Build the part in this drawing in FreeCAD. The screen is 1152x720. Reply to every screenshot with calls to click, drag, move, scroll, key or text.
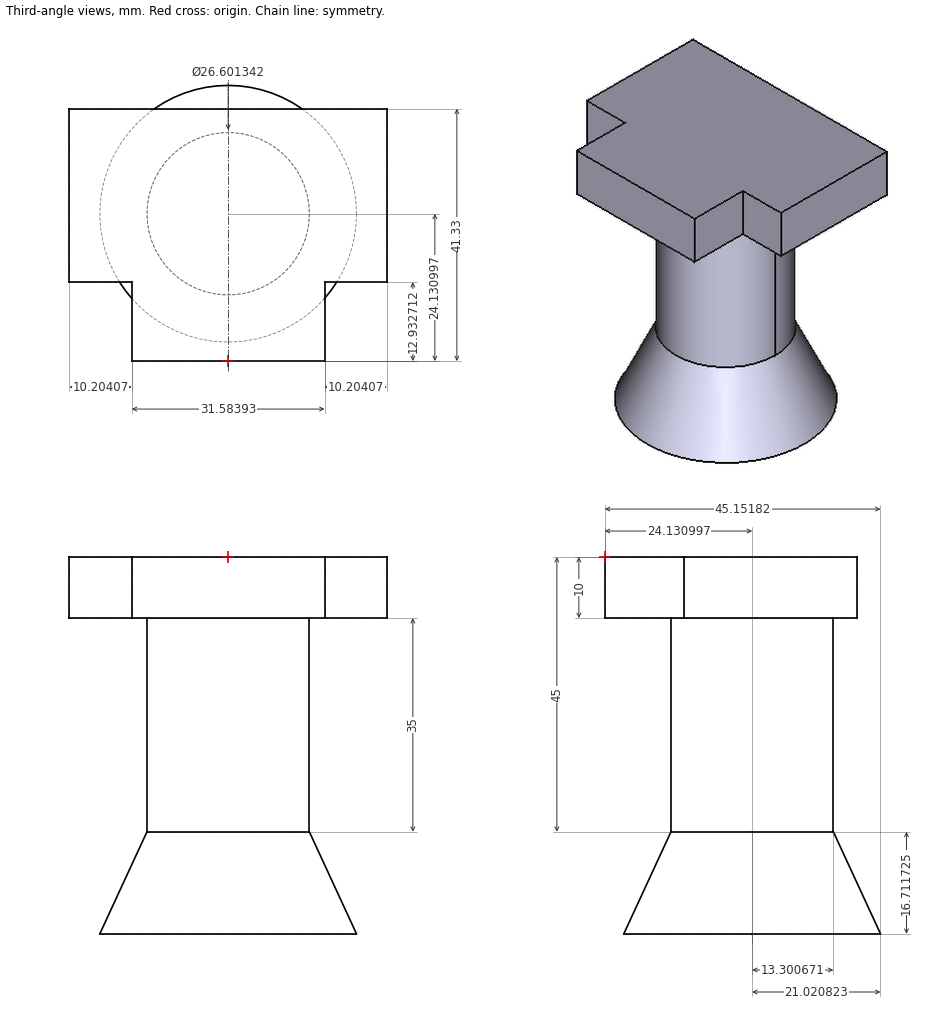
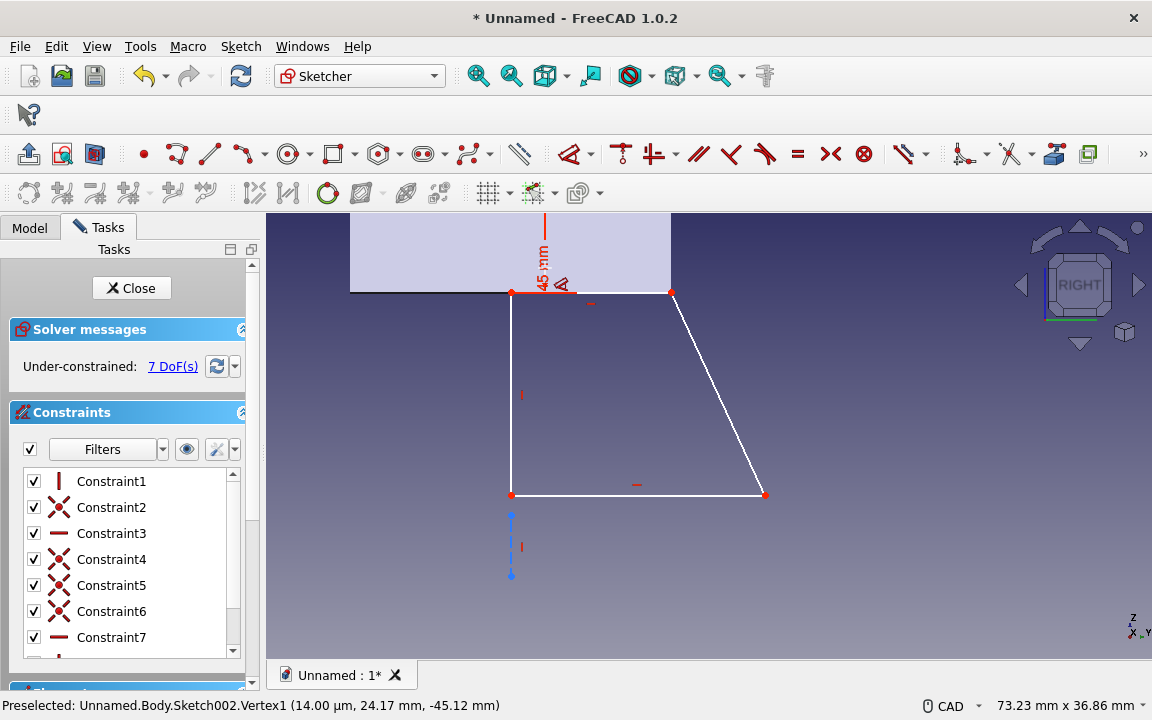
click(511, 354)
click(477, 394)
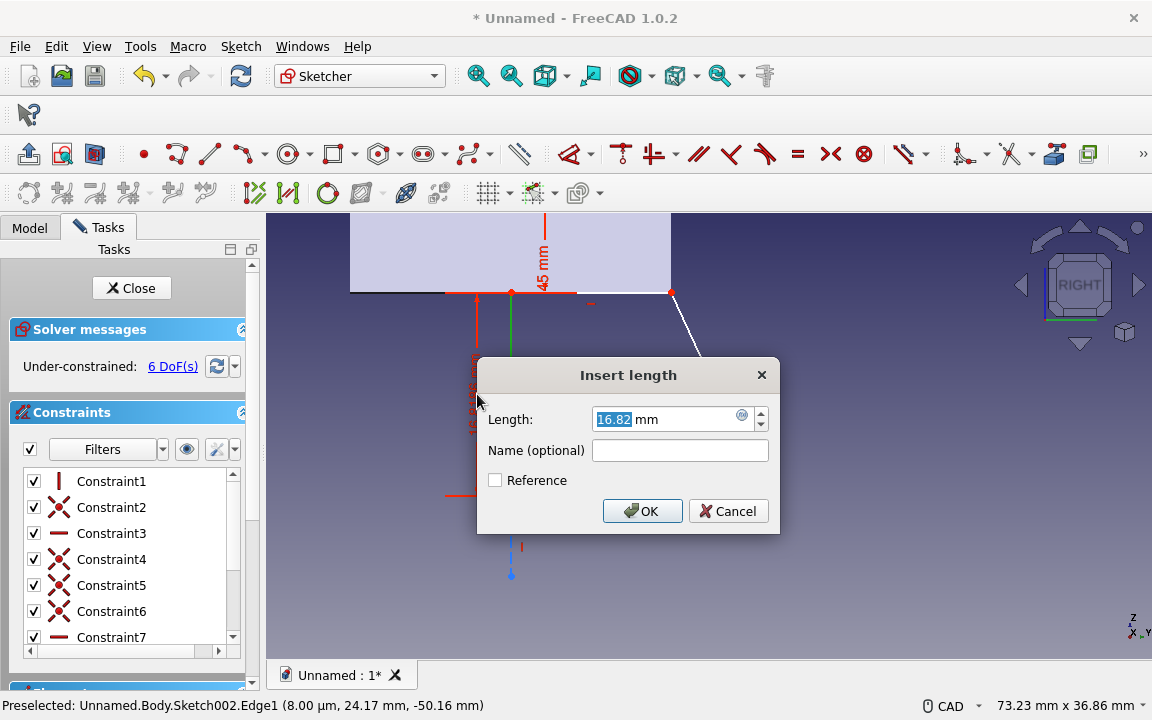
text(16.711725)
key(Return)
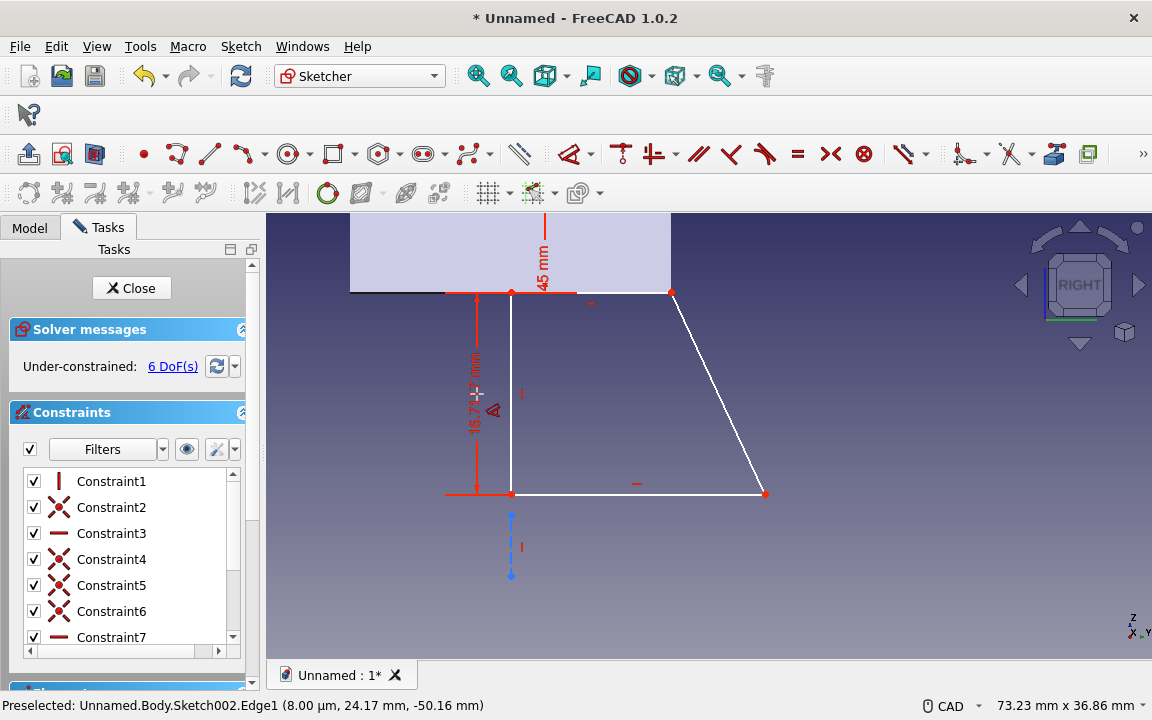
click(587, 495)
click(638, 529)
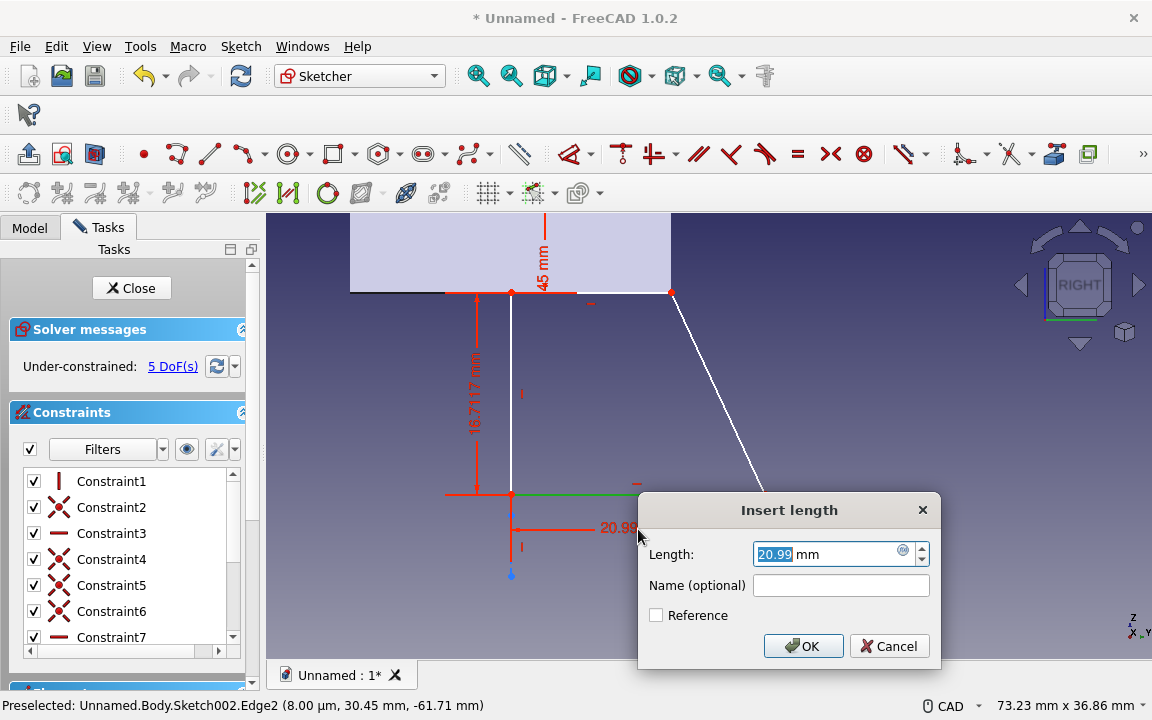
text(21.020823)
key(Return)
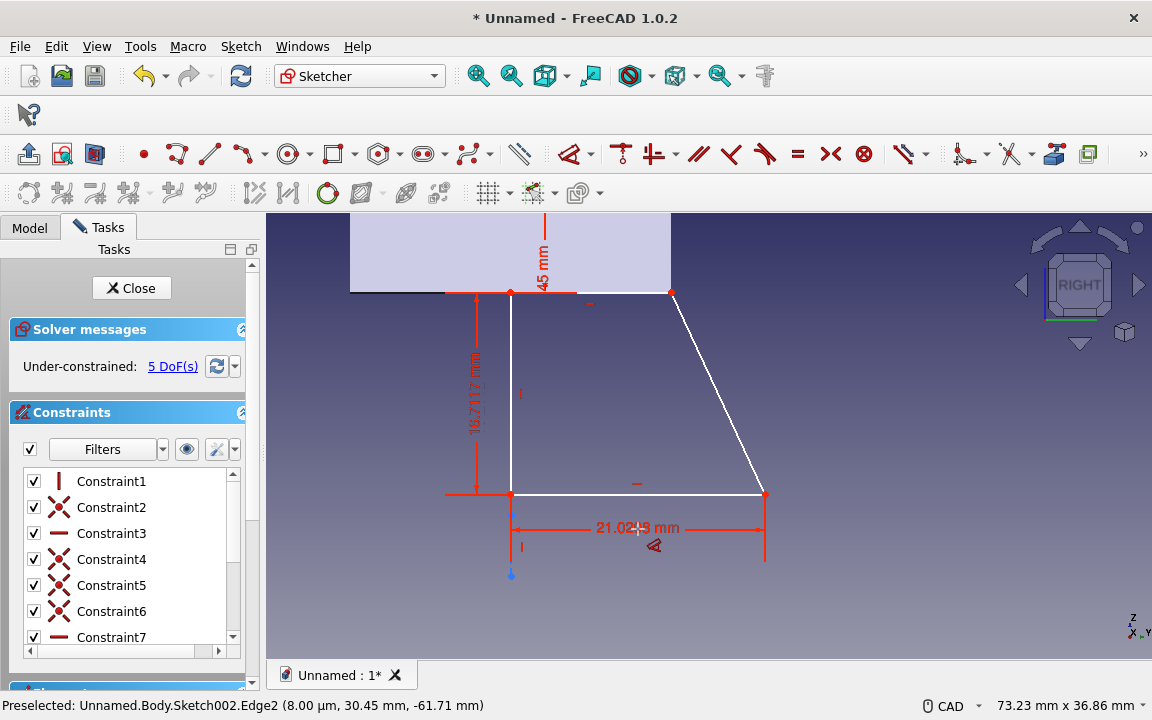
click(623, 293)
click(628, 259)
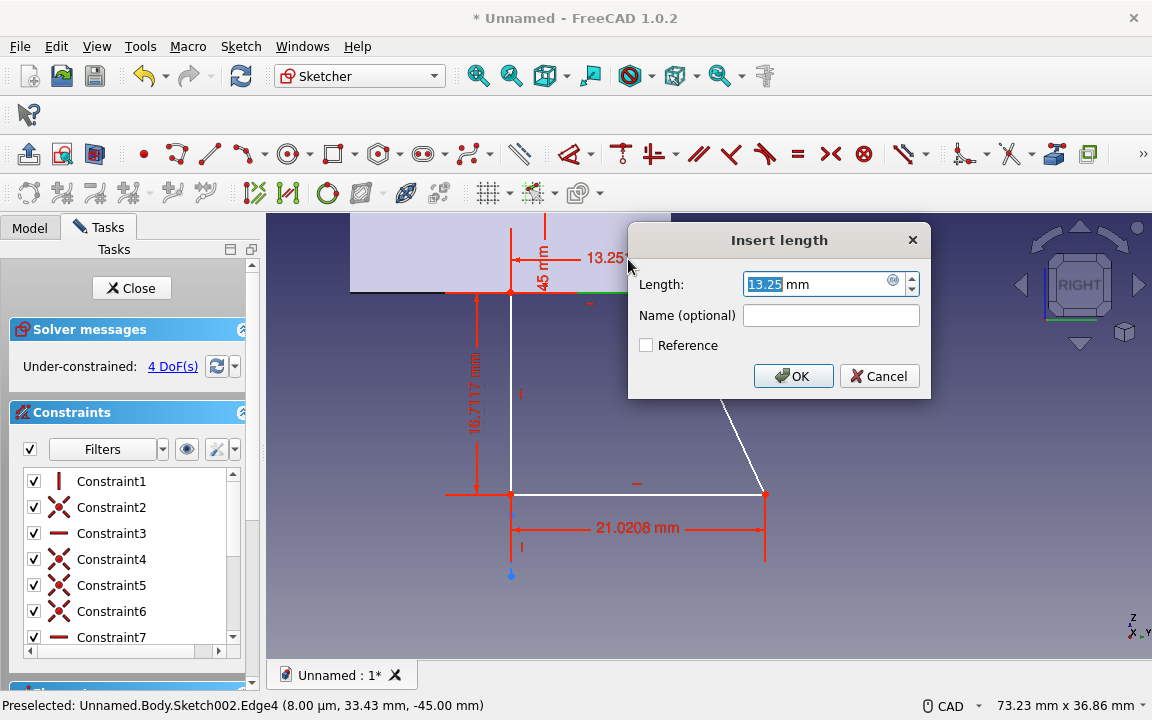
text(13.300671)
key(Return)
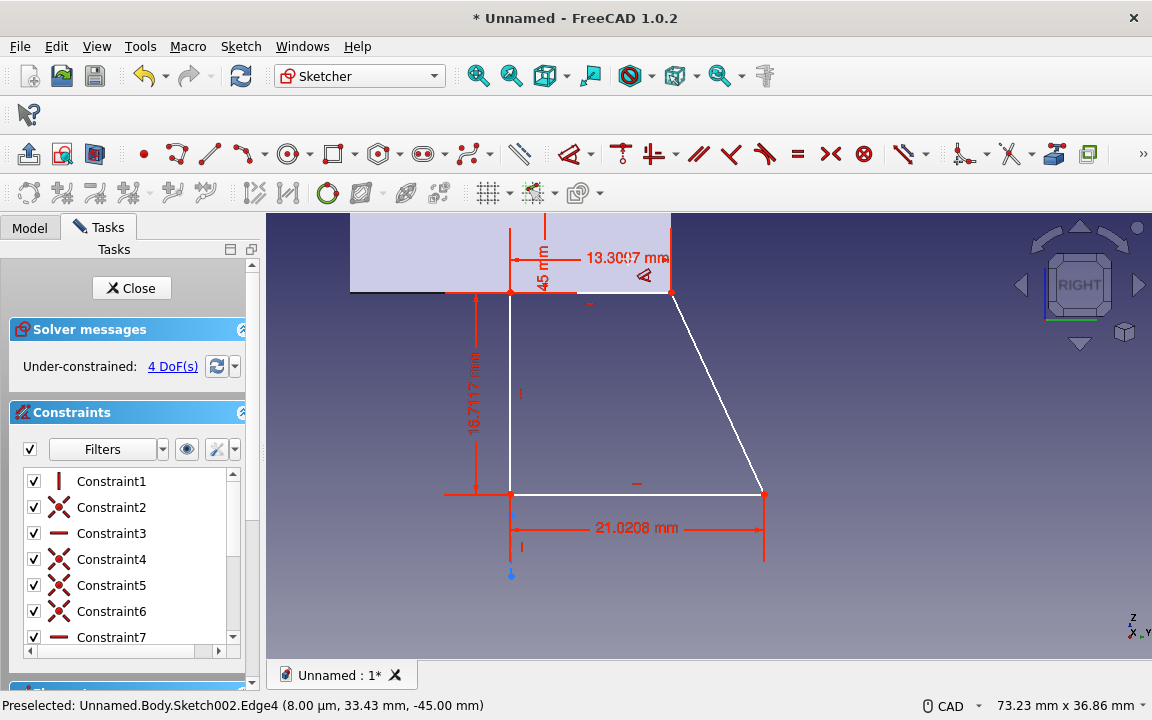
click(764, 495)
click(529, 529)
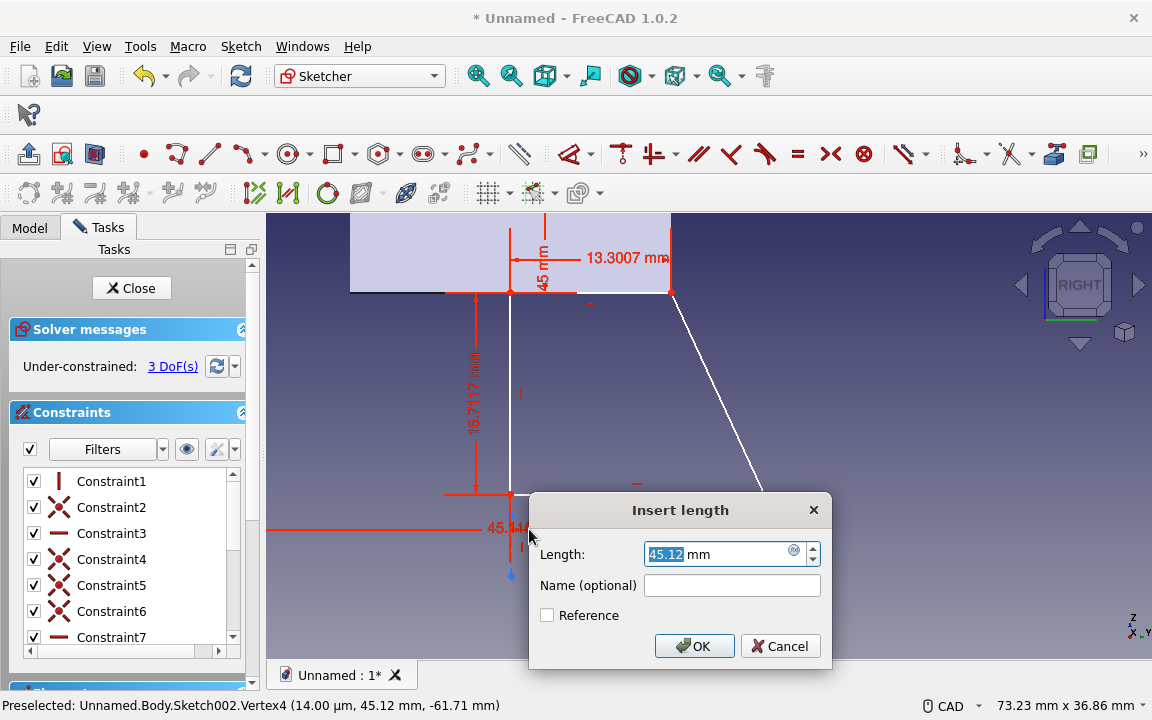
text(45.15182)
key(Return)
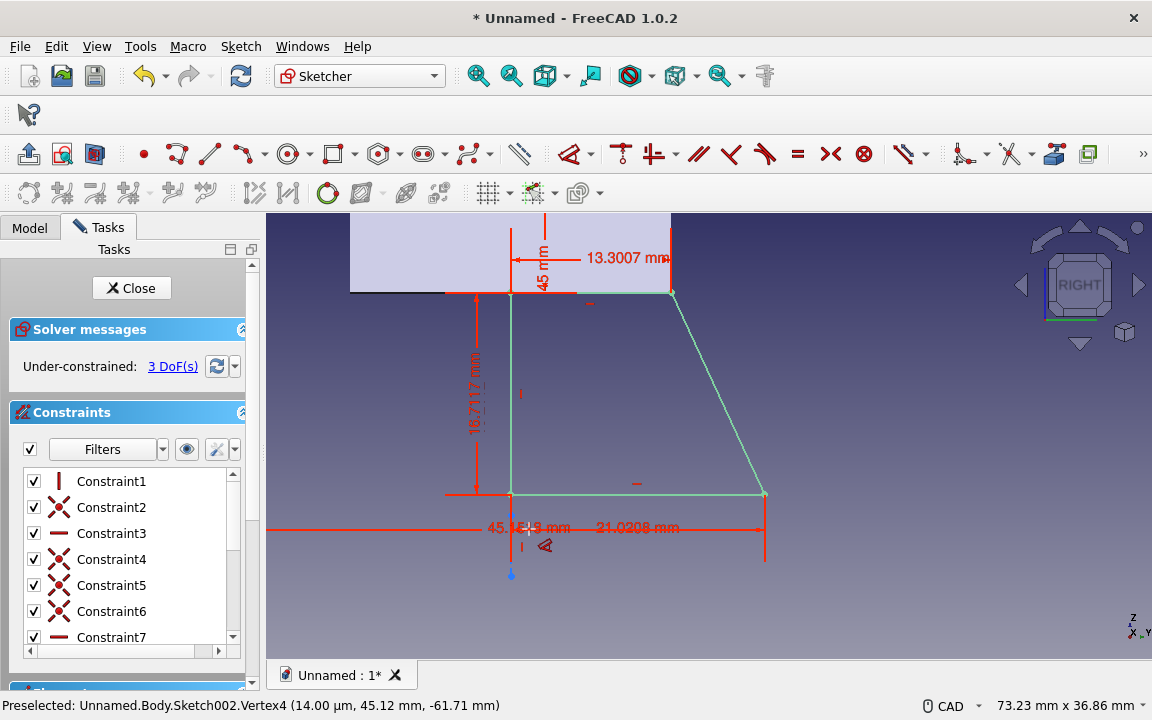
click(511, 516)
click(403, 550)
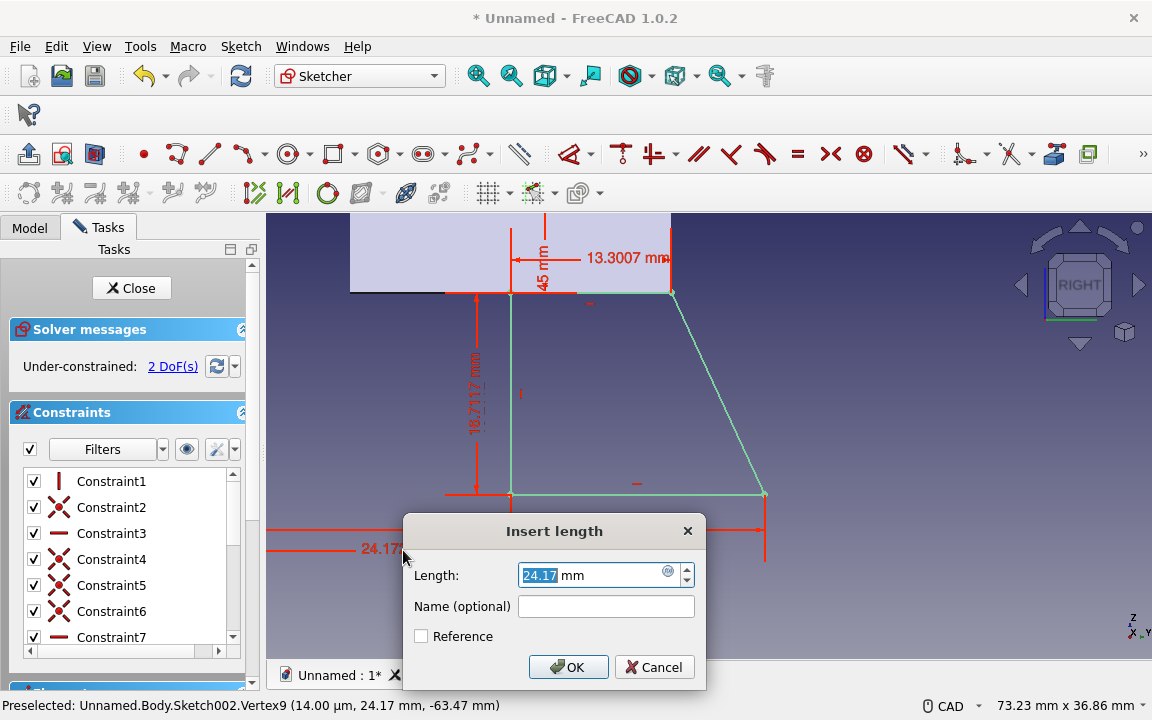
text(24.130997)
key(Return)
key(Escape)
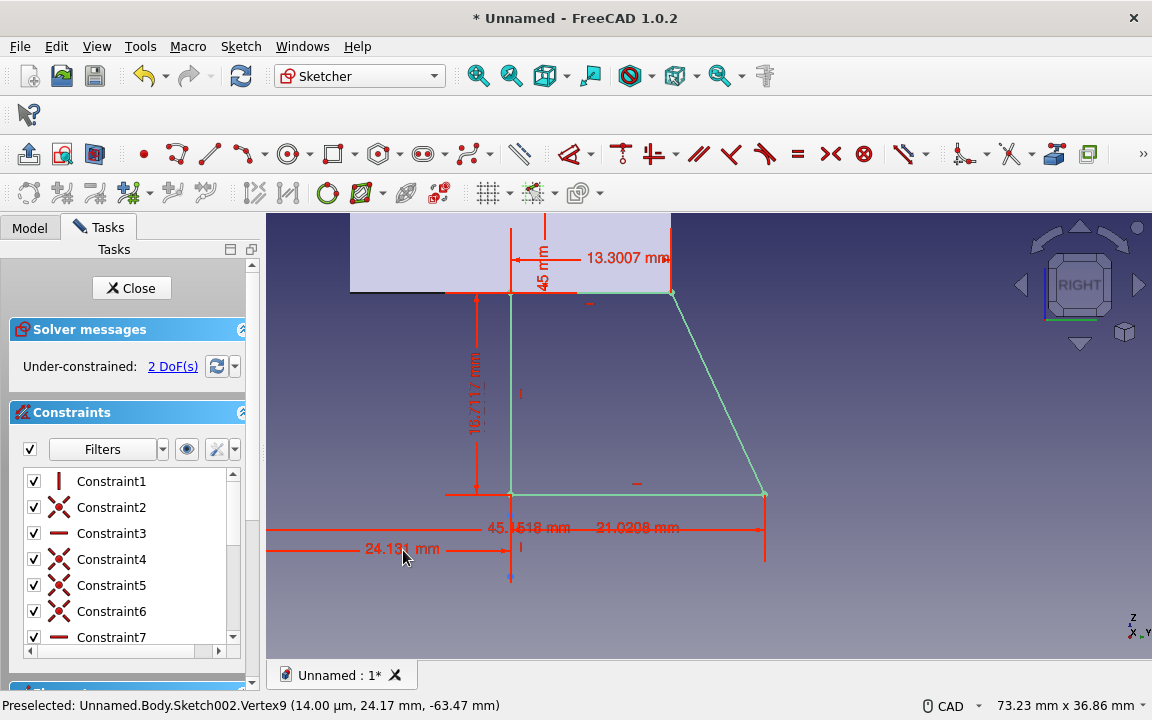
click(132, 288)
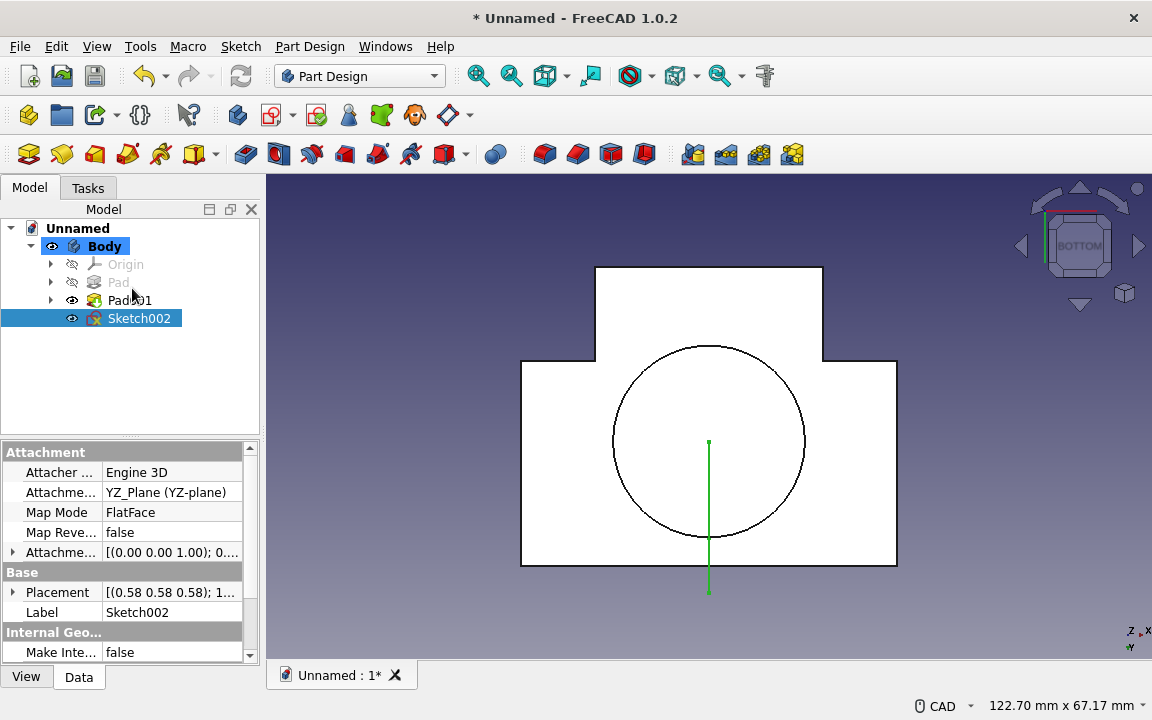
click(62, 154)